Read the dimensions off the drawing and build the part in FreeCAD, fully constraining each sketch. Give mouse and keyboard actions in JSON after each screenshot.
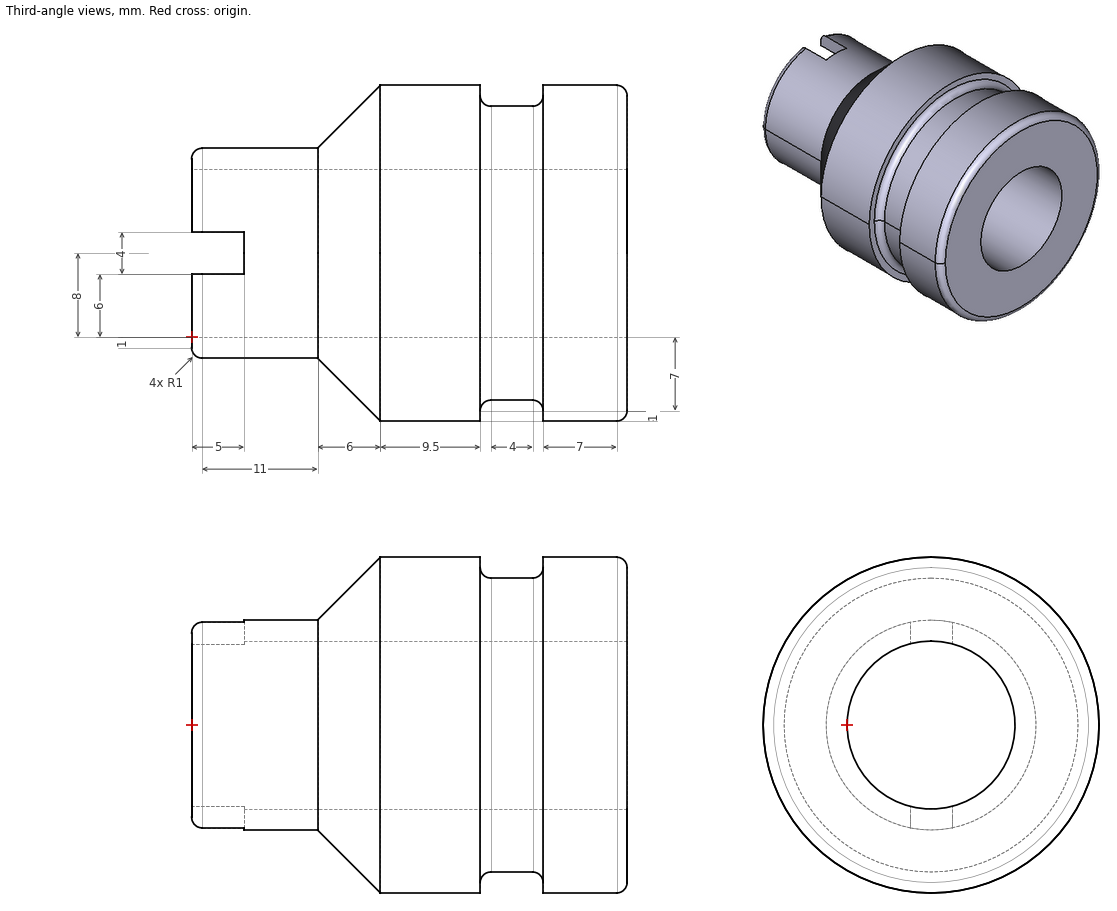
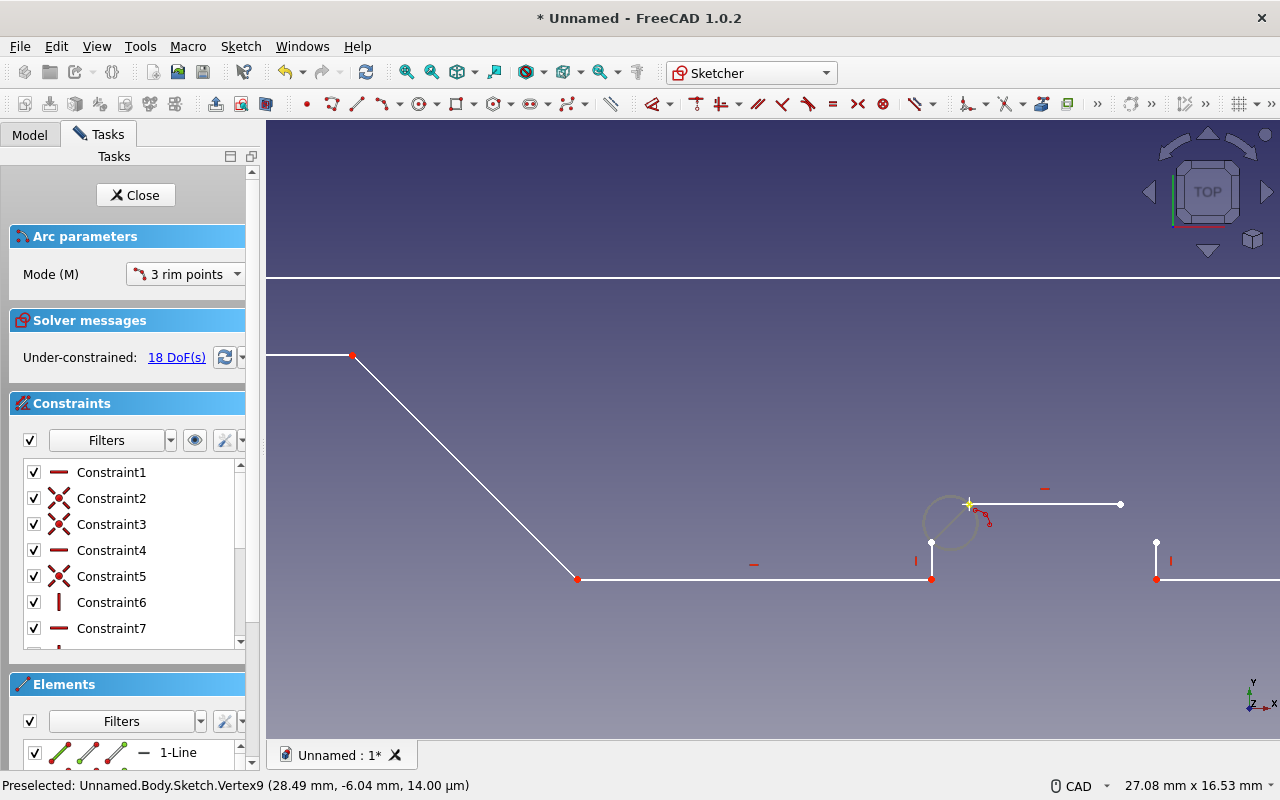
{"action": "scroll", "coordinate": [943, 514], "scroll_direction": "up", "scroll_amount": 2}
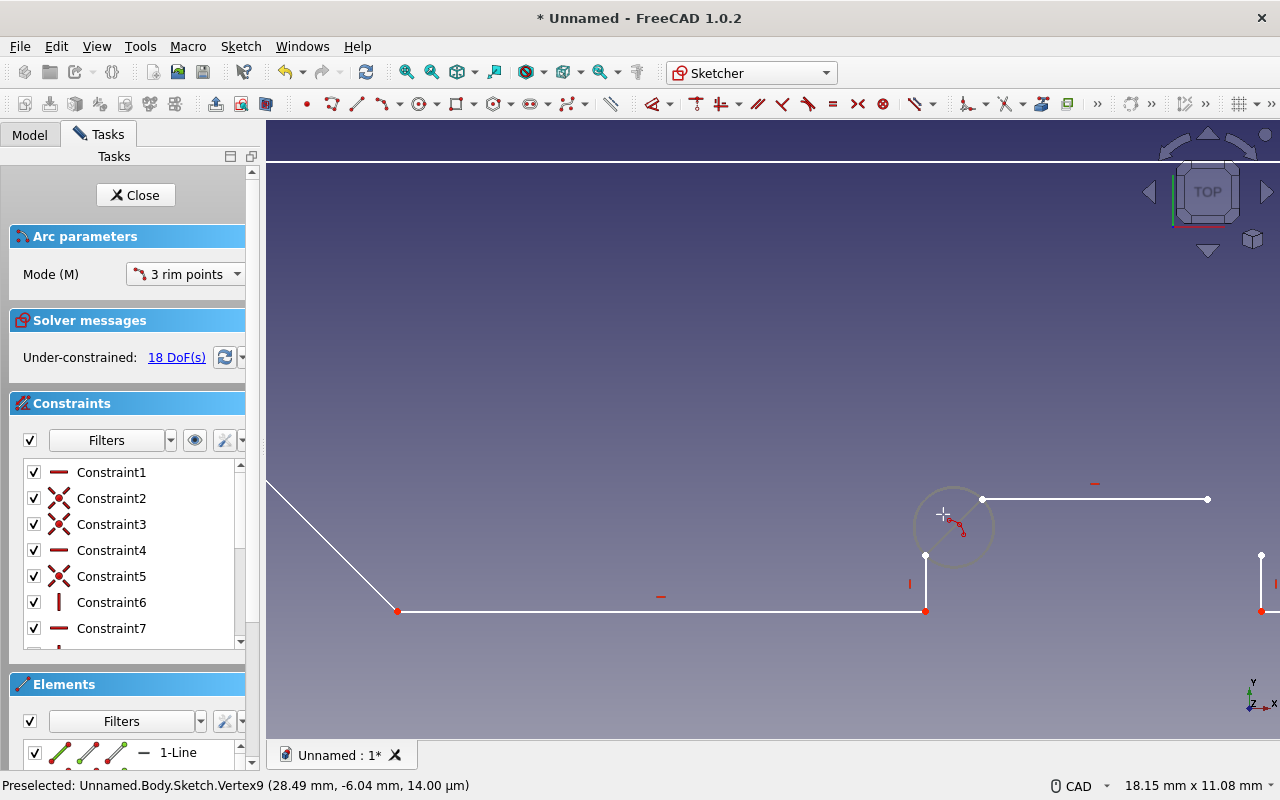
{"action": "left_click", "coordinate": [943, 513]}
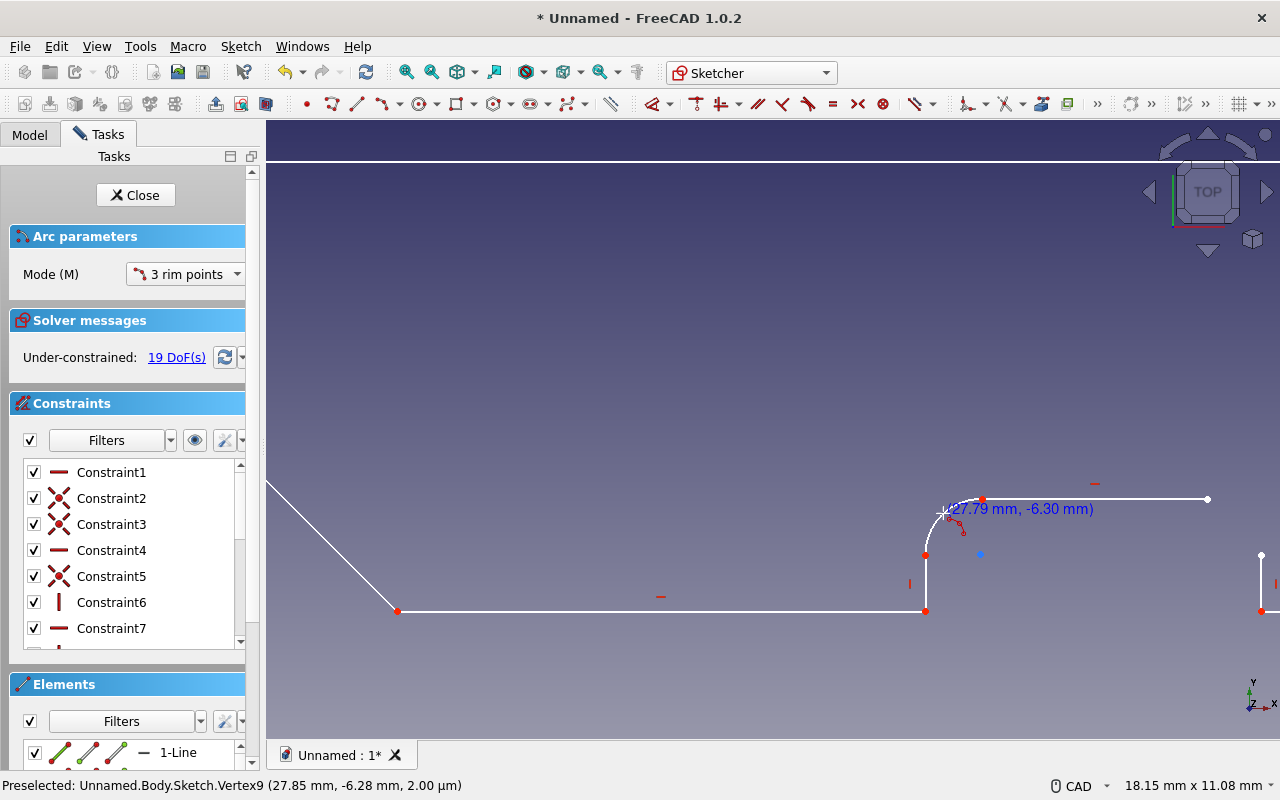
{"action": "scroll", "coordinate": [744, 497], "scroll_direction": "down", "scroll_amount": 8}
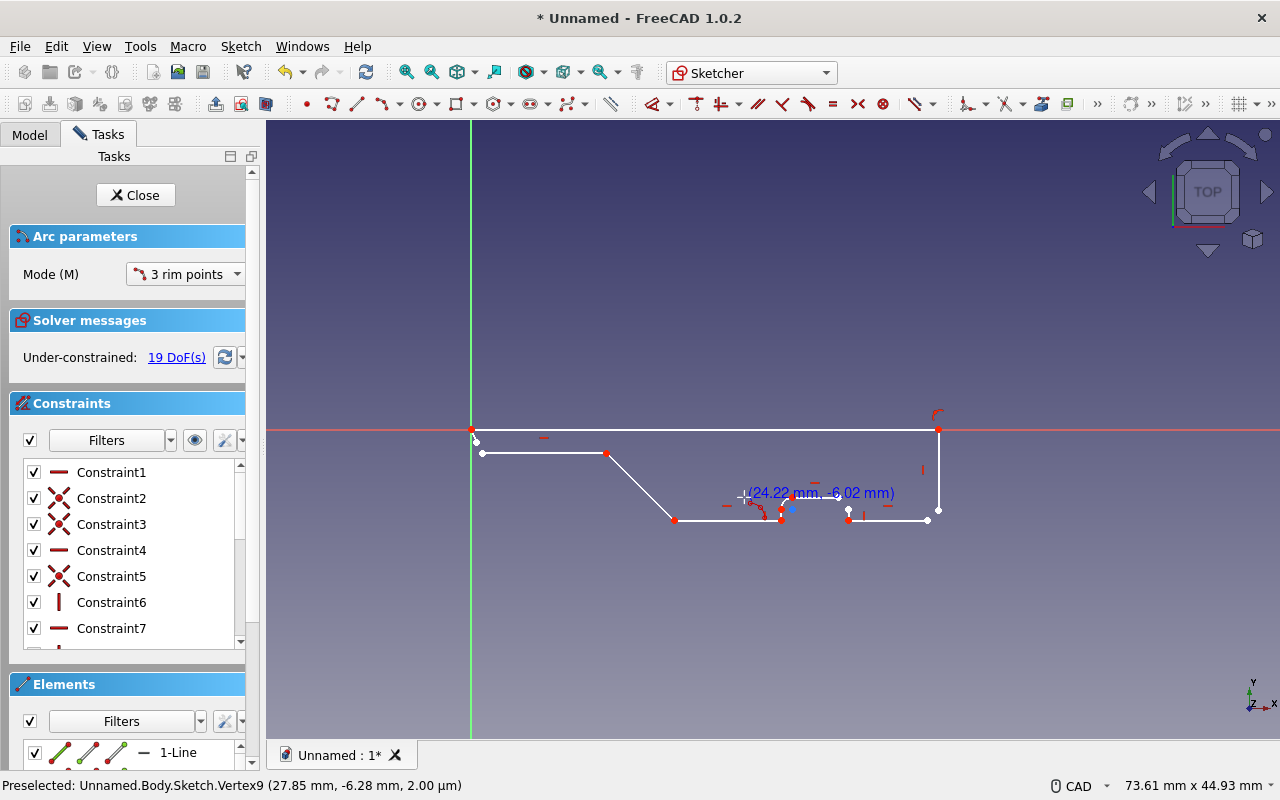
{"action": "left_click", "coordinate": [838, 498]}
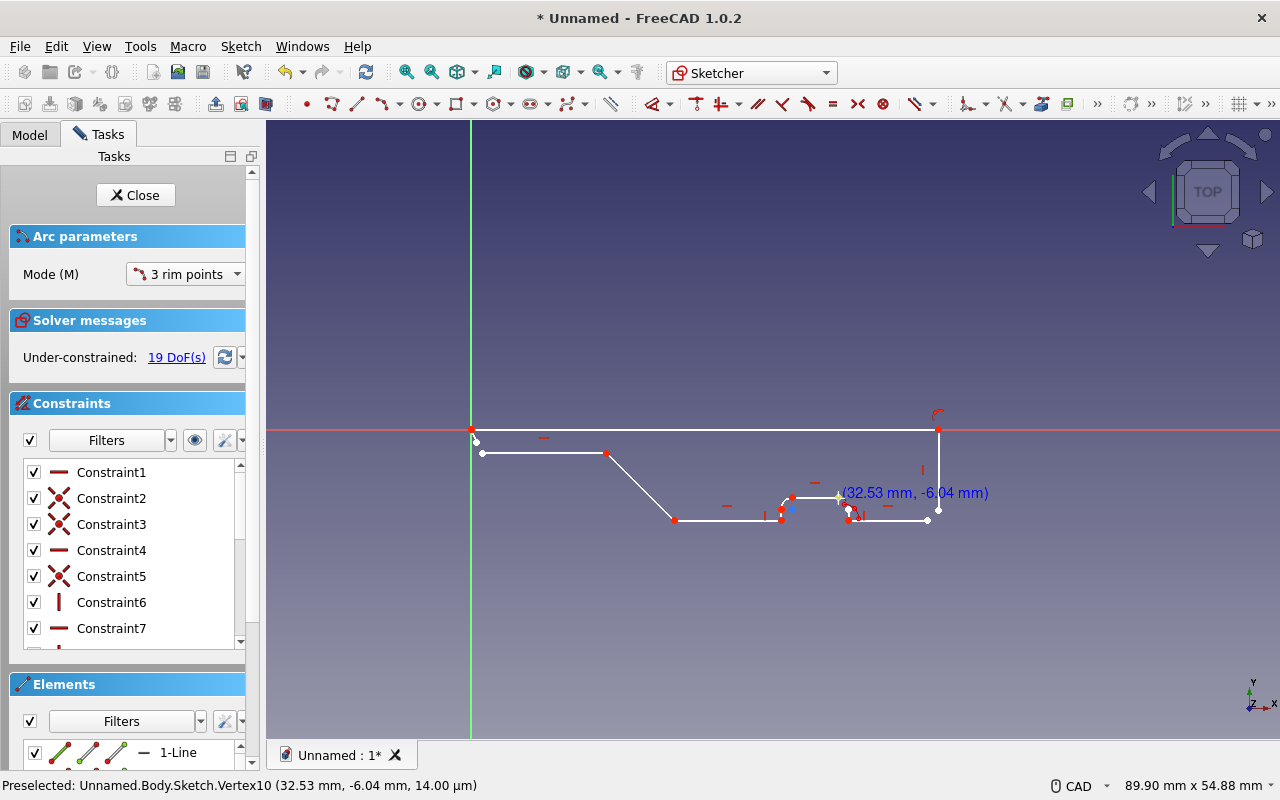
{"action": "scroll", "coordinate": [849, 509], "scroll_direction": "up", "scroll_amount": 6}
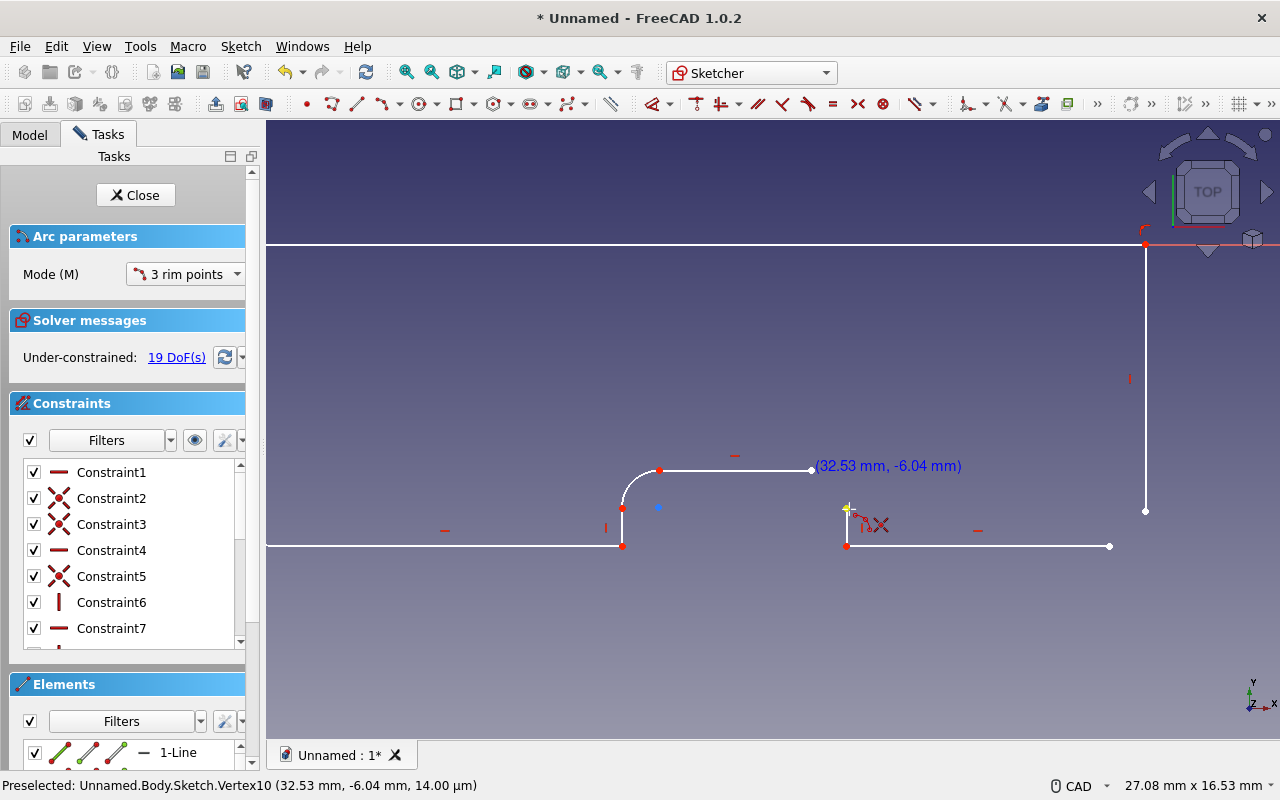
{"action": "left_click", "coordinate": [847, 509]}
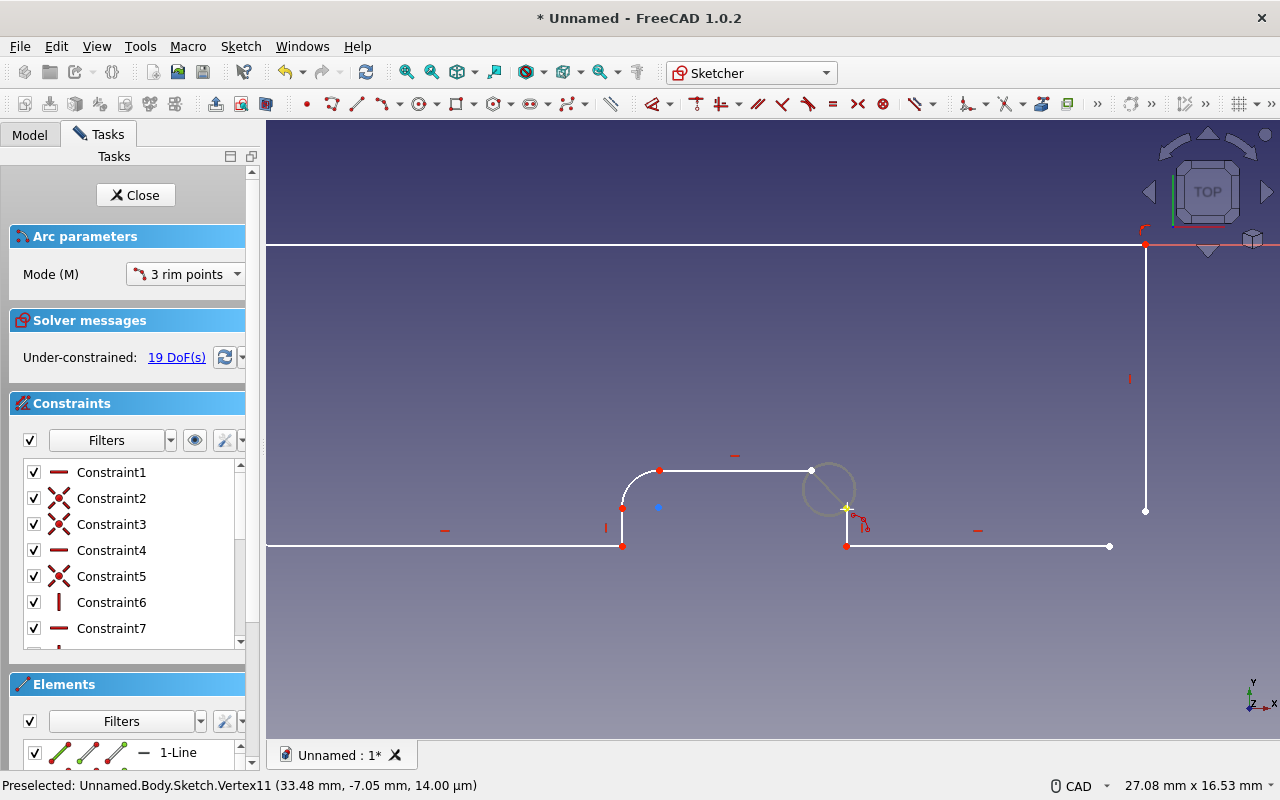
{"action": "scroll", "coordinate": [837, 480], "scroll_direction": "up", "scroll_amount": 2}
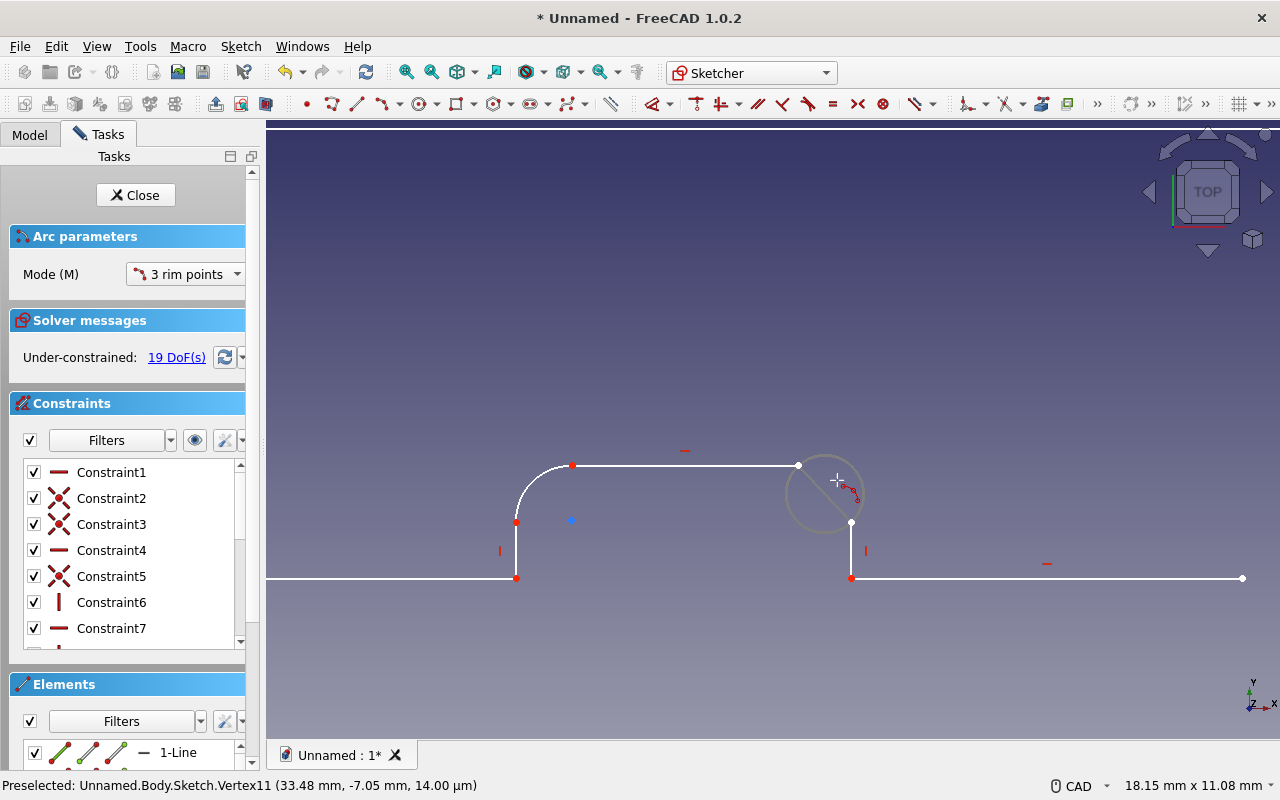
{"action": "left_click", "coordinate": [836, 480]}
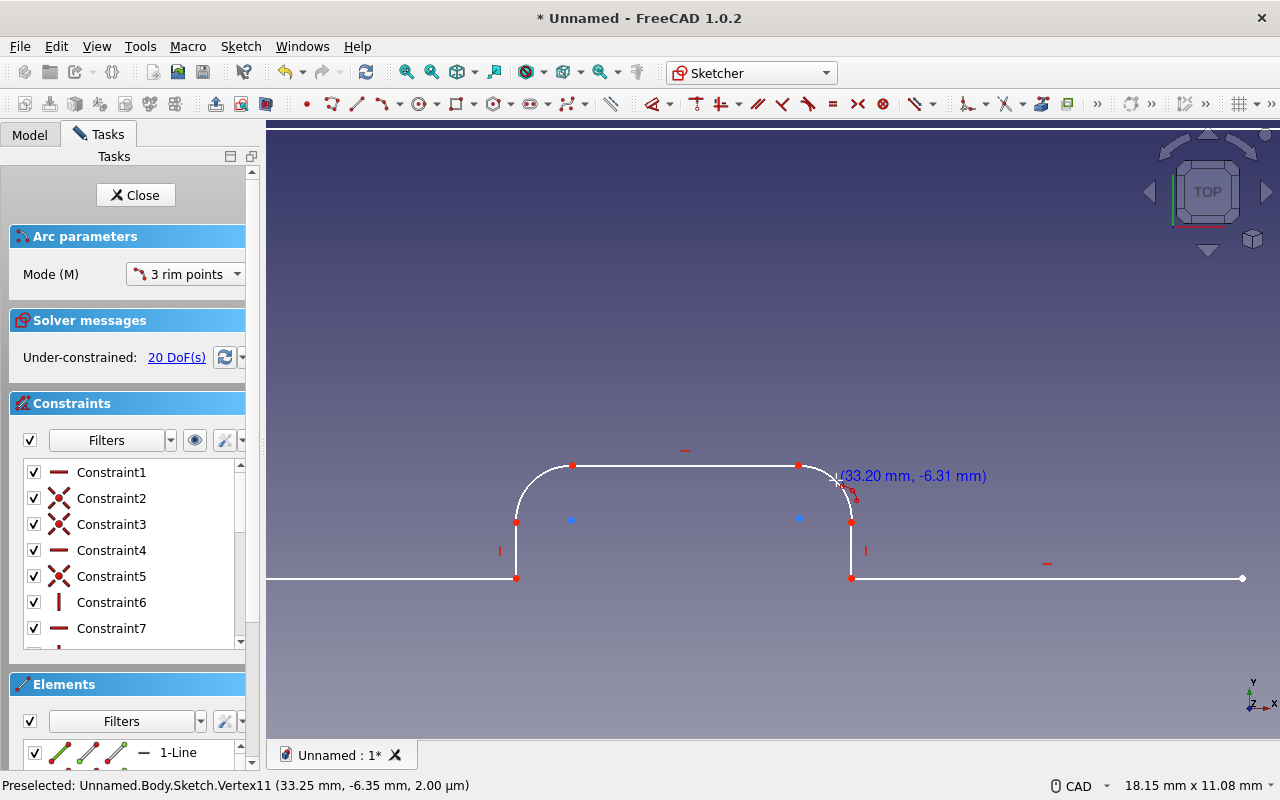
{"action": "scroll", "coordinate": [847, 506], "scroll_direction": "down", "scroll_amount": 8}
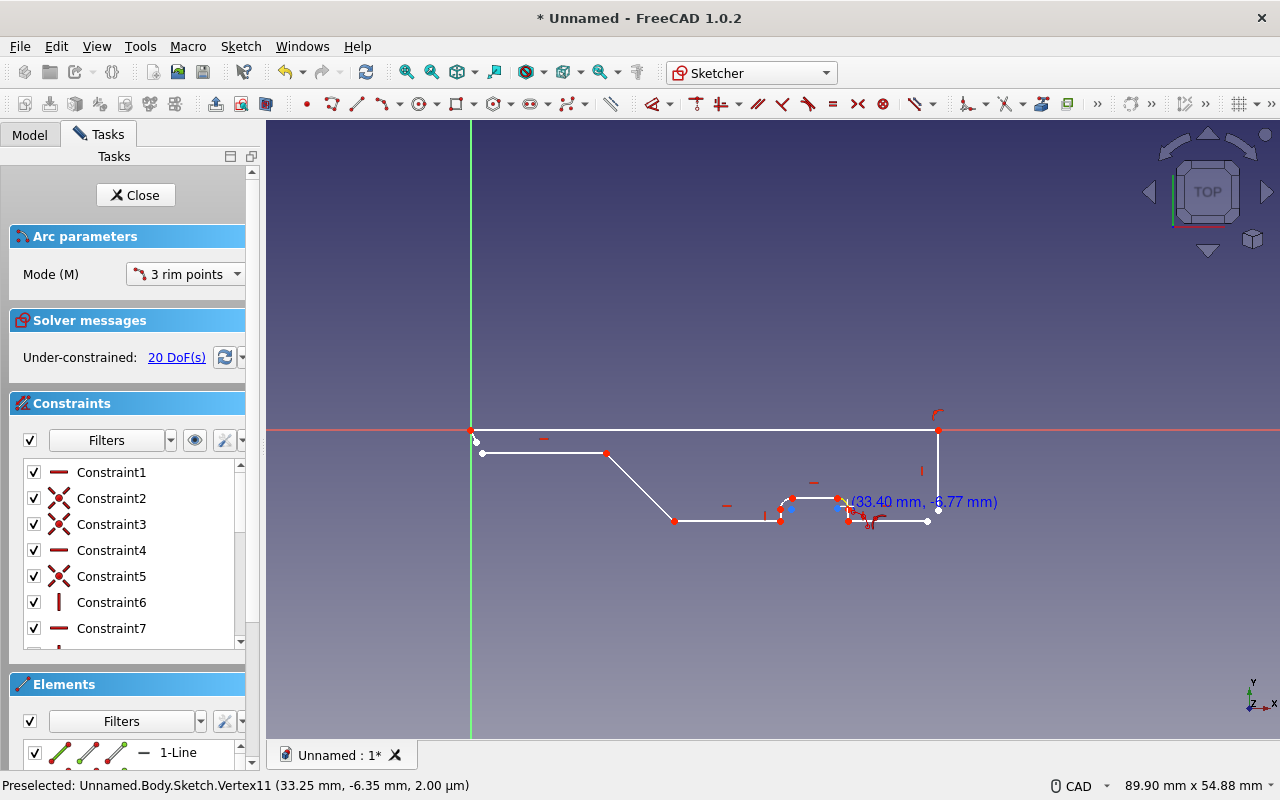
{"action": "left_click", "coordinate": [927, 521]}
{"action": "left_click", "coordinate": [938, 511]}